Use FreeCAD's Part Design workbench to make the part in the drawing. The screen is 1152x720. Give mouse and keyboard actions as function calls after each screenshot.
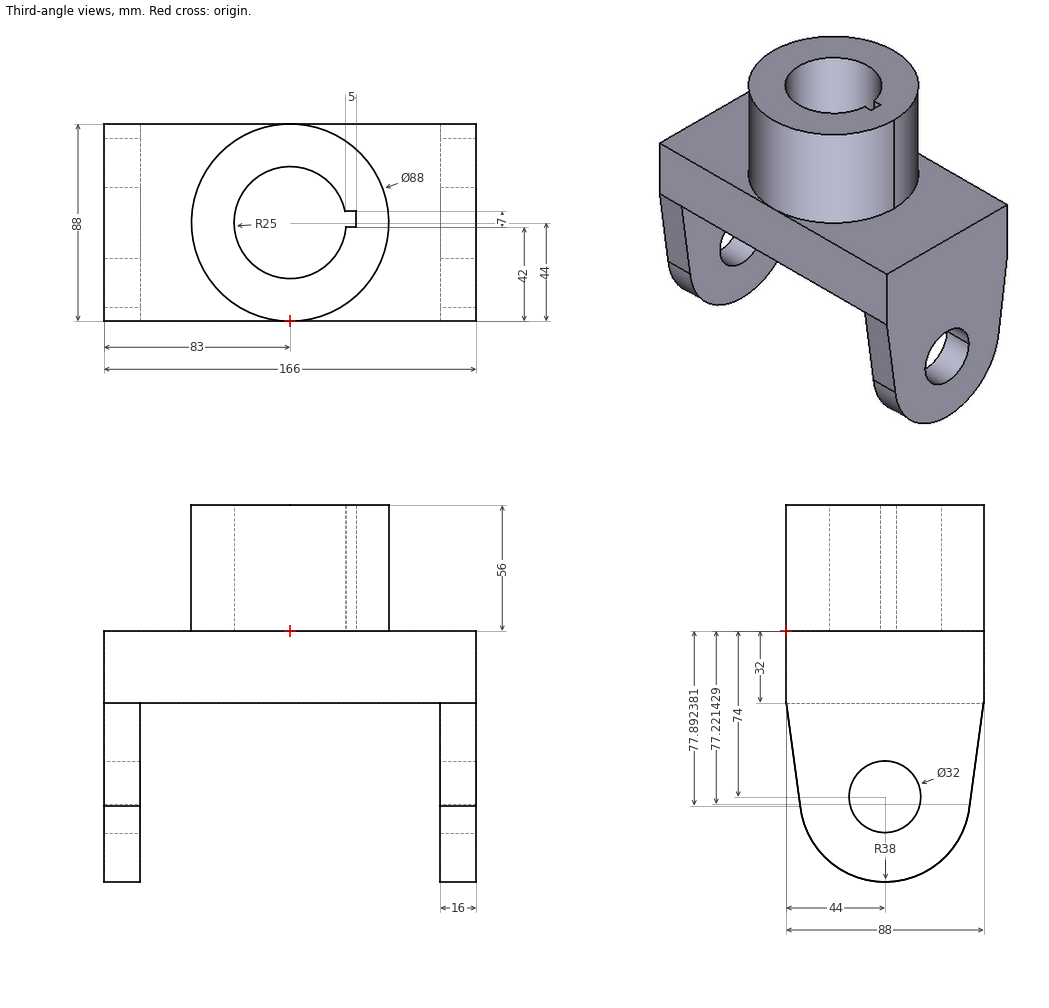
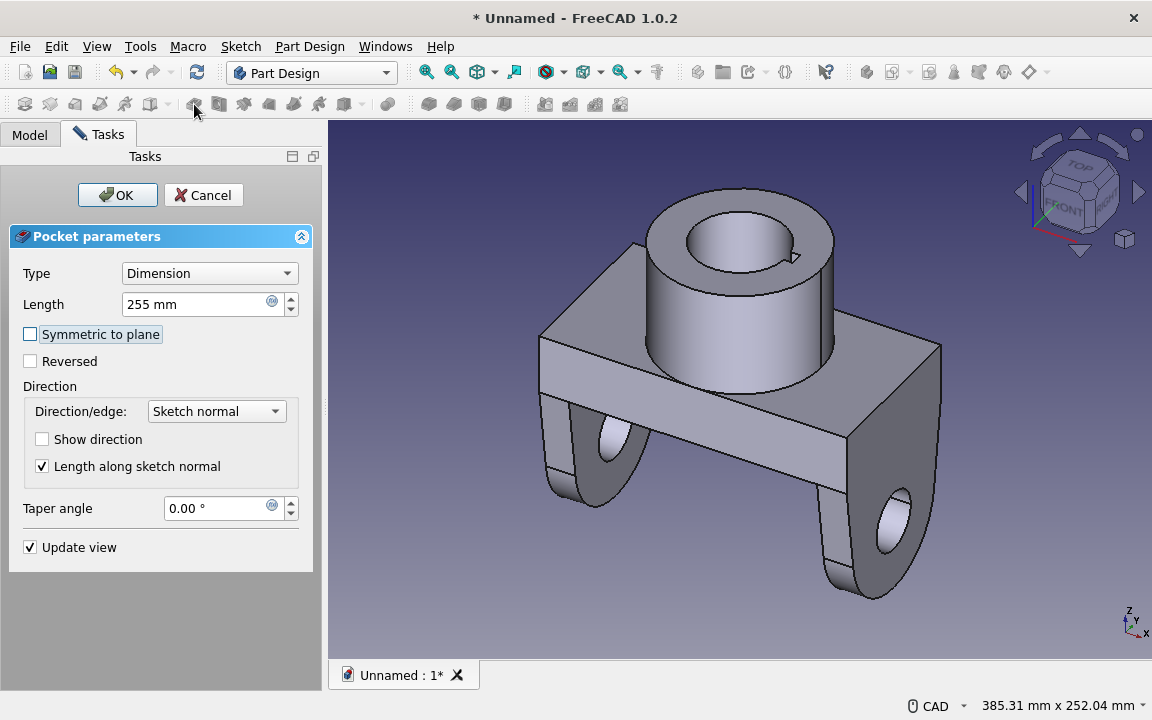
click(118, 195)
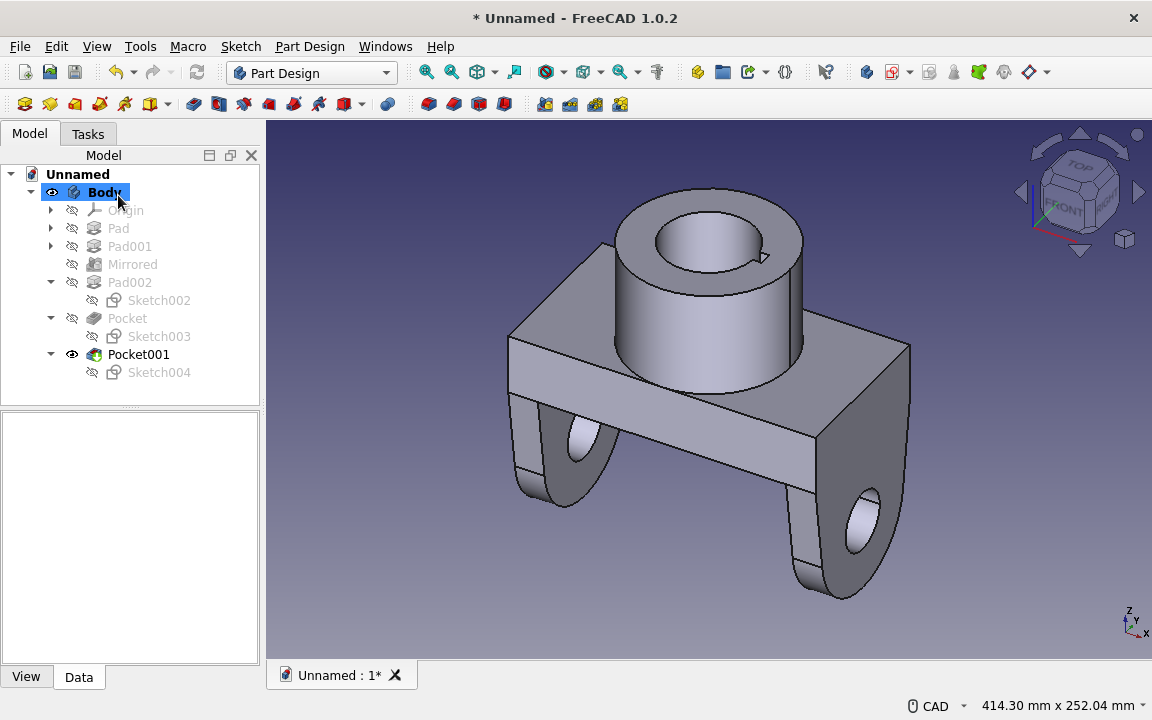
key(0)